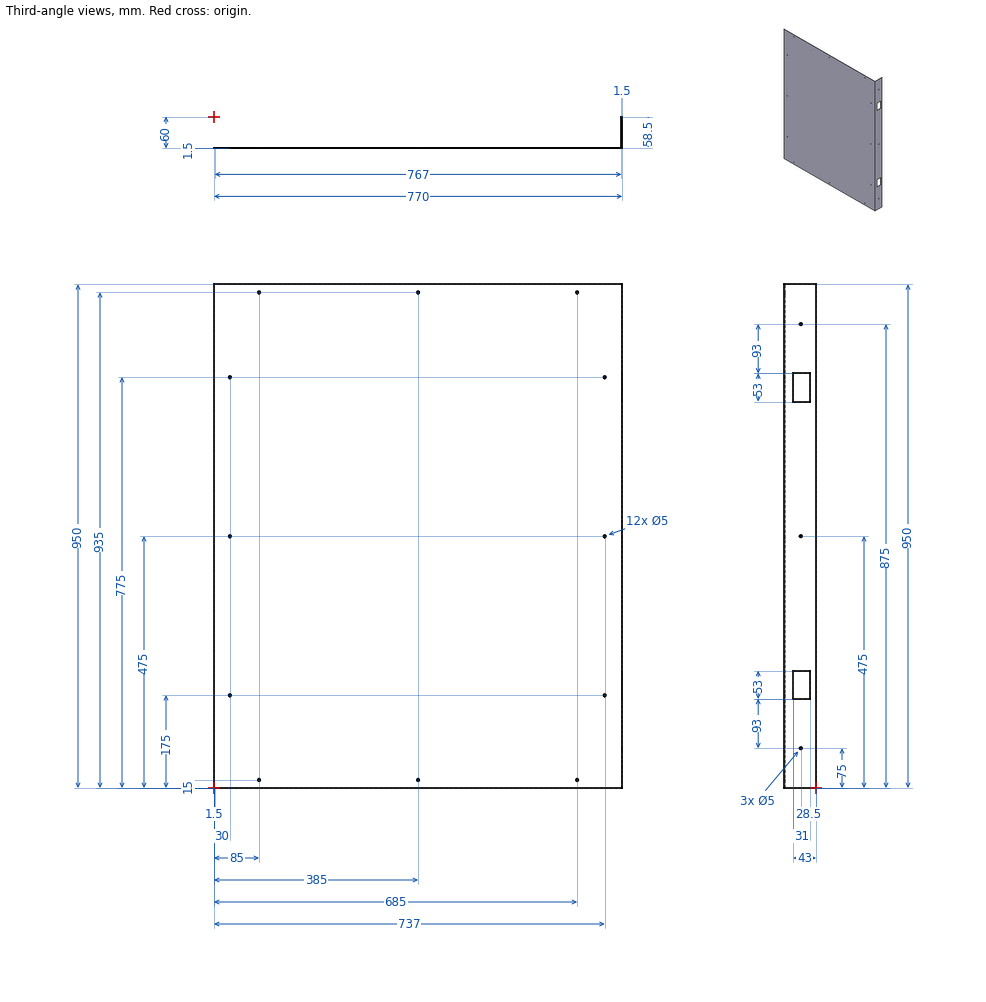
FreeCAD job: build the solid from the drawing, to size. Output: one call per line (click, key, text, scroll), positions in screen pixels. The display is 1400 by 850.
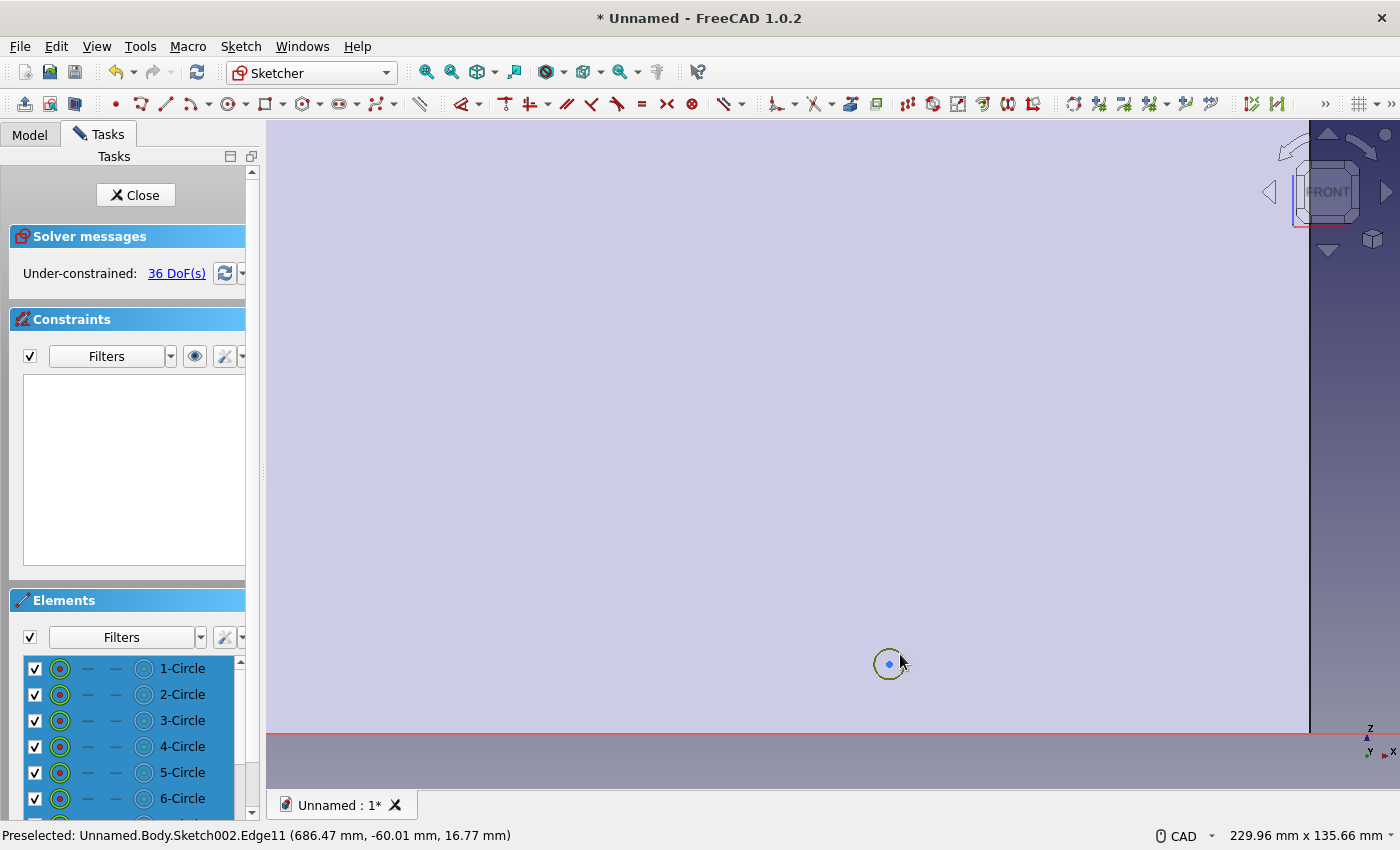
scroll(907, 657, down, 12)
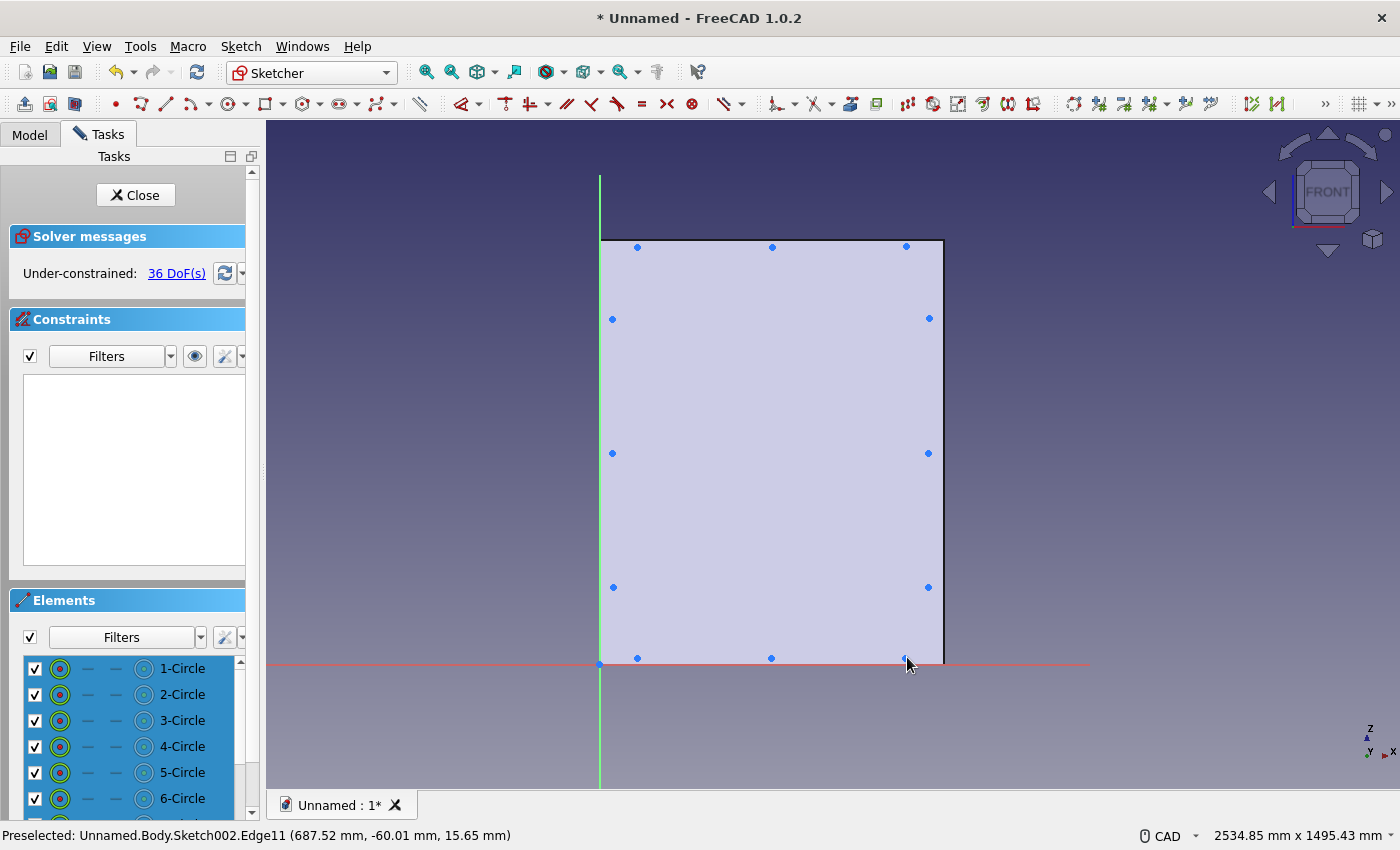
scroll(773, 657, up, 12)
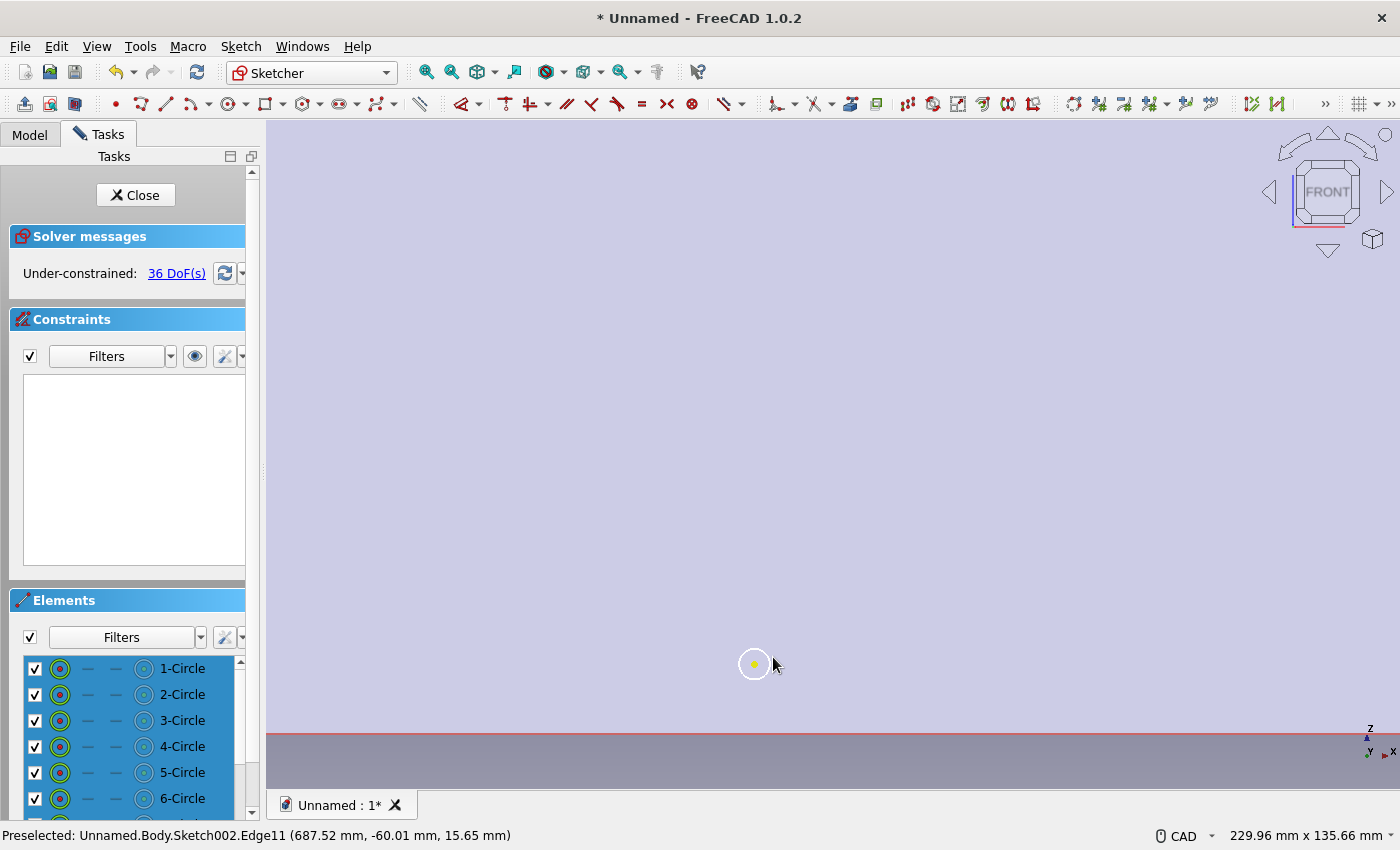
click(765, 653)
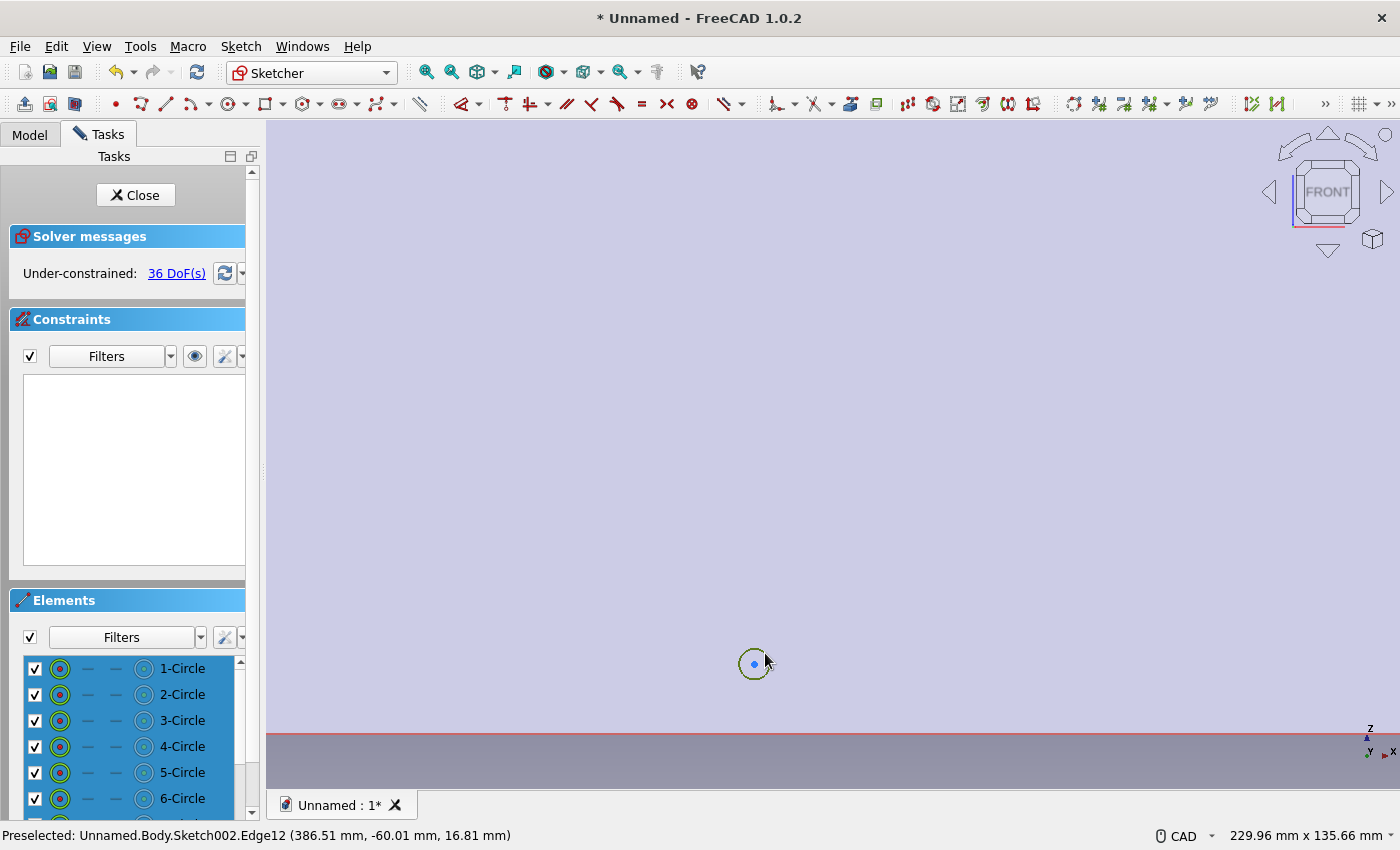
click(642, 104)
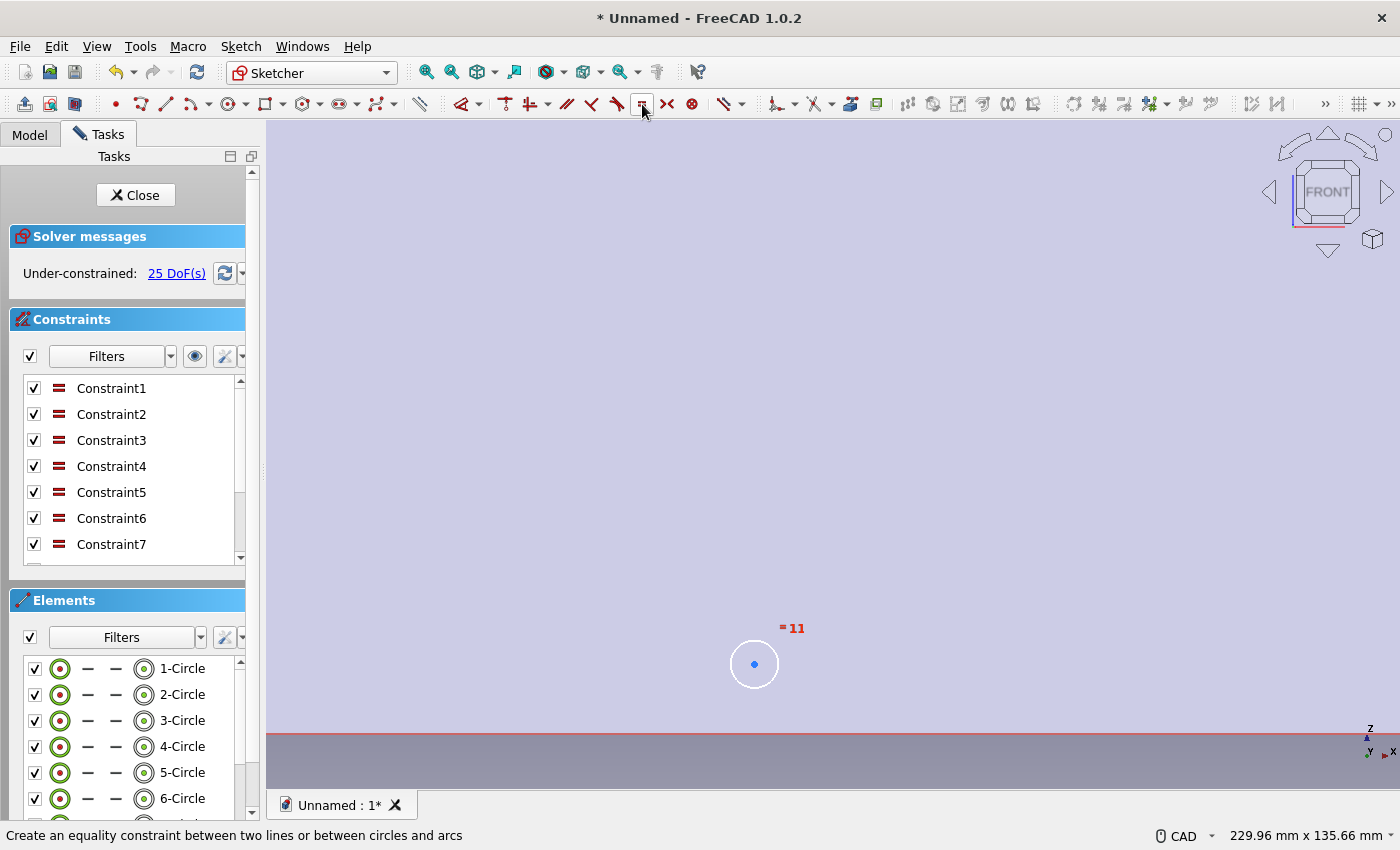
click(460, 104)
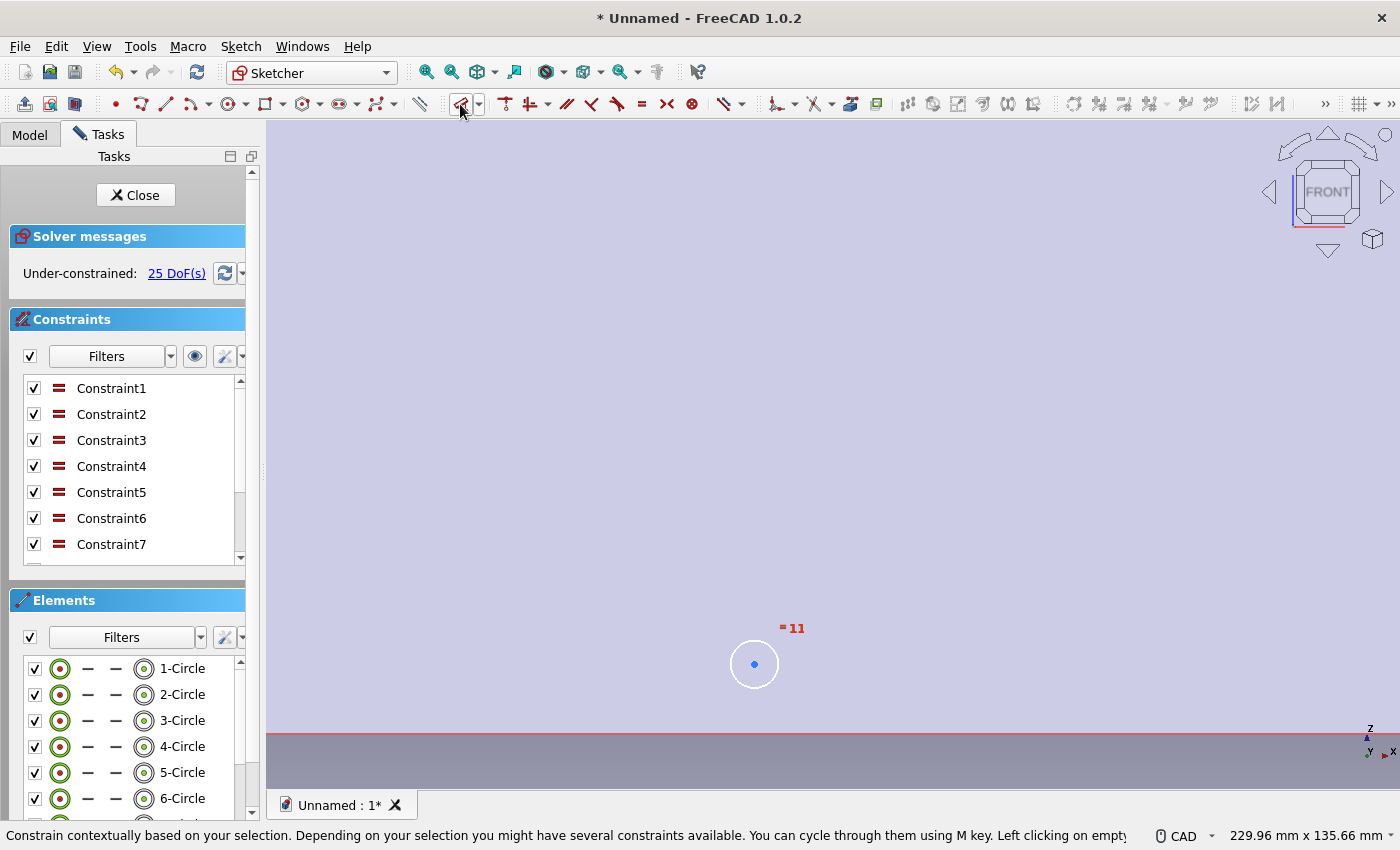
scroll(773, 657, down, 12)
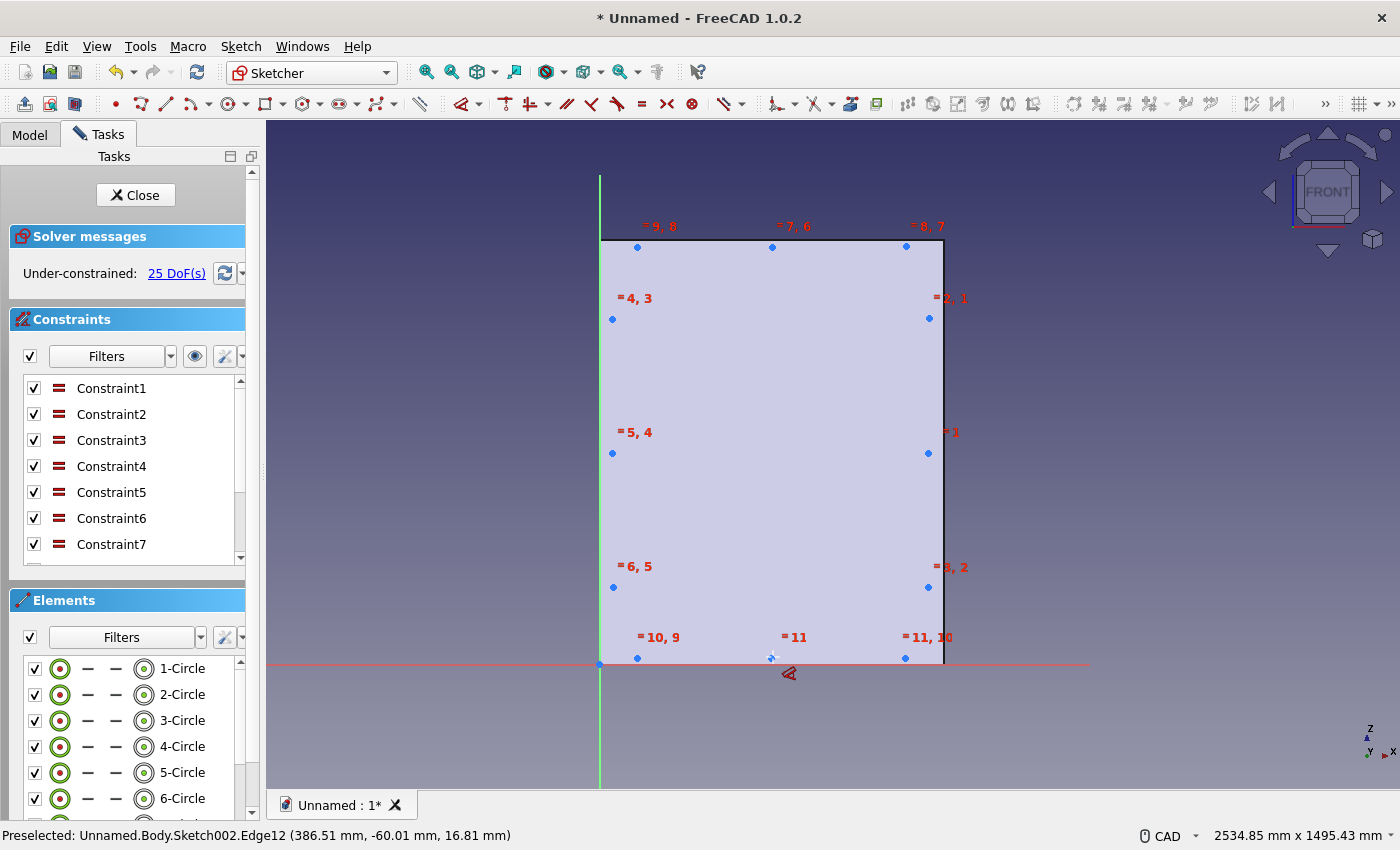
scroll(930, 452, up, 15)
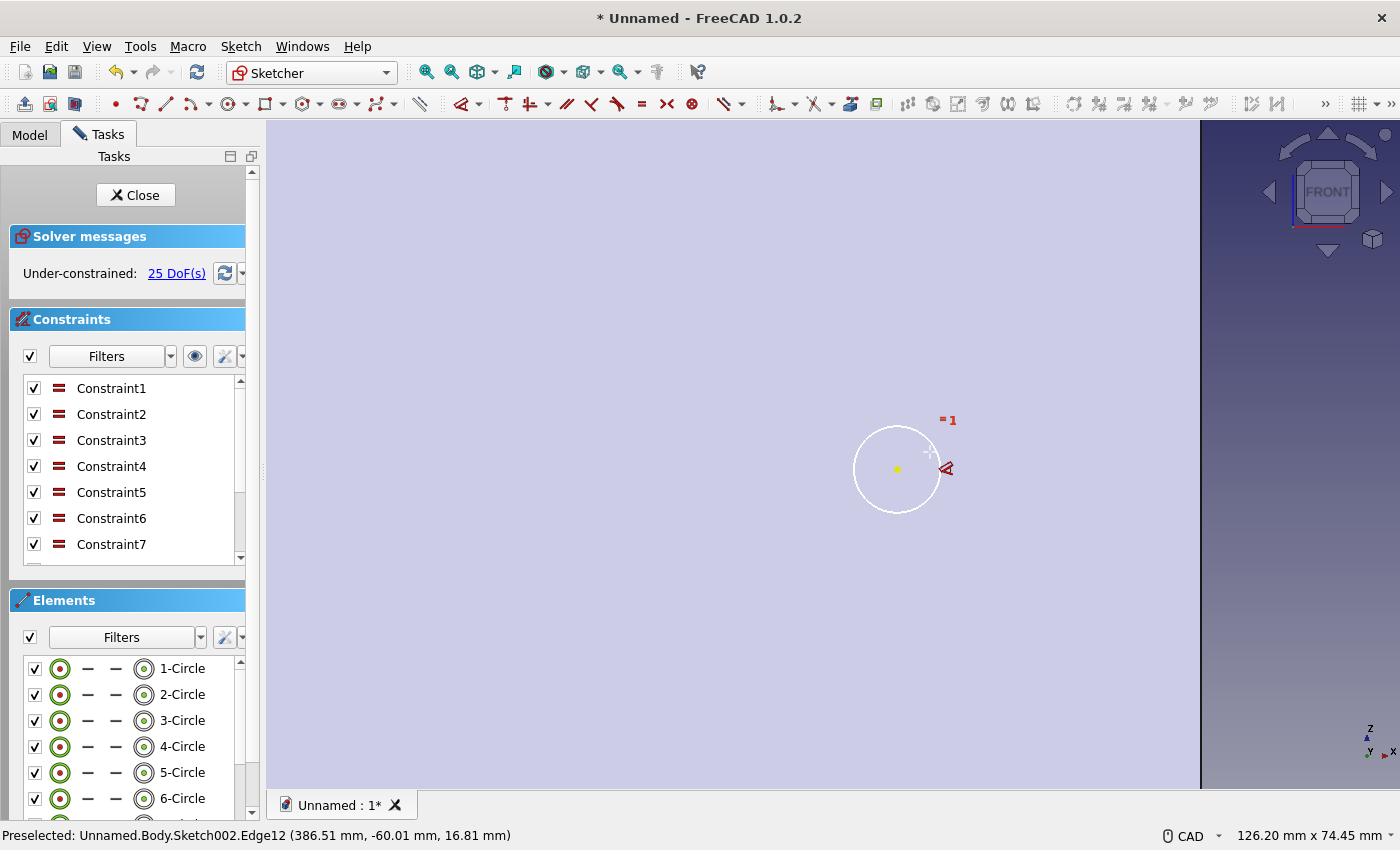
click(928, 439)
click(951, 416)